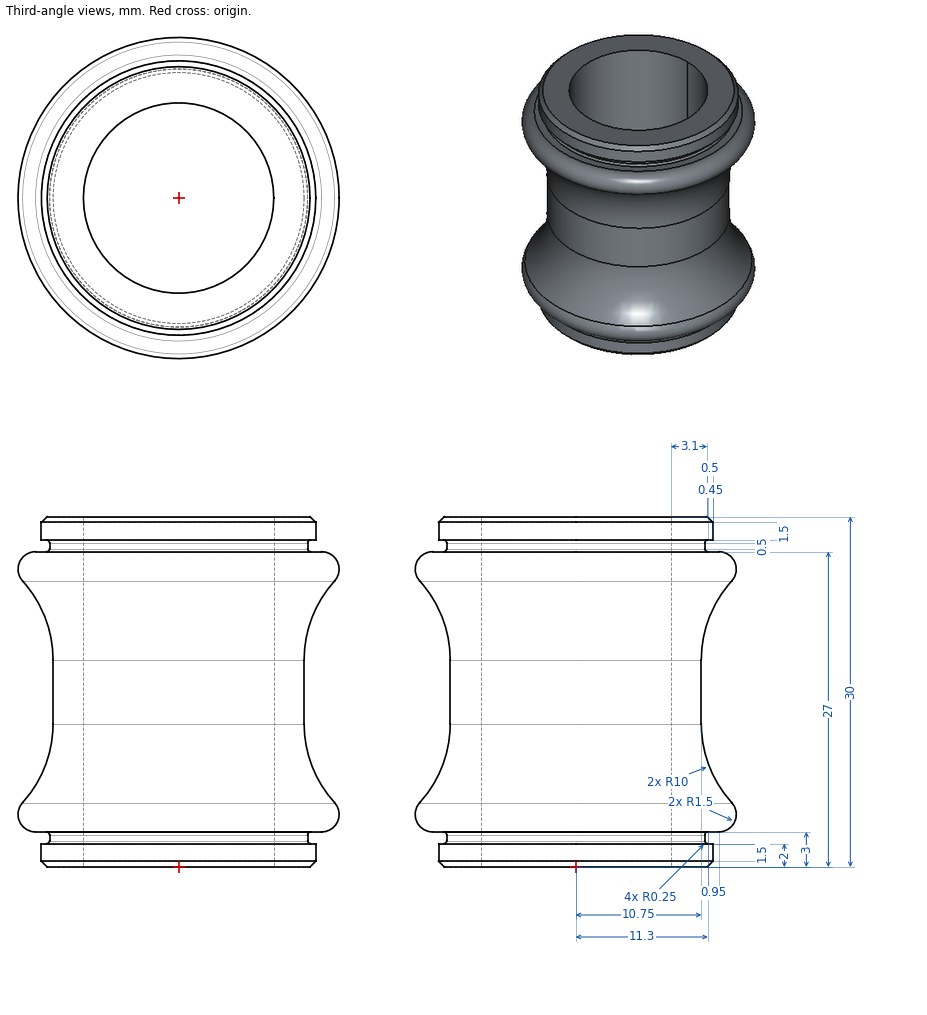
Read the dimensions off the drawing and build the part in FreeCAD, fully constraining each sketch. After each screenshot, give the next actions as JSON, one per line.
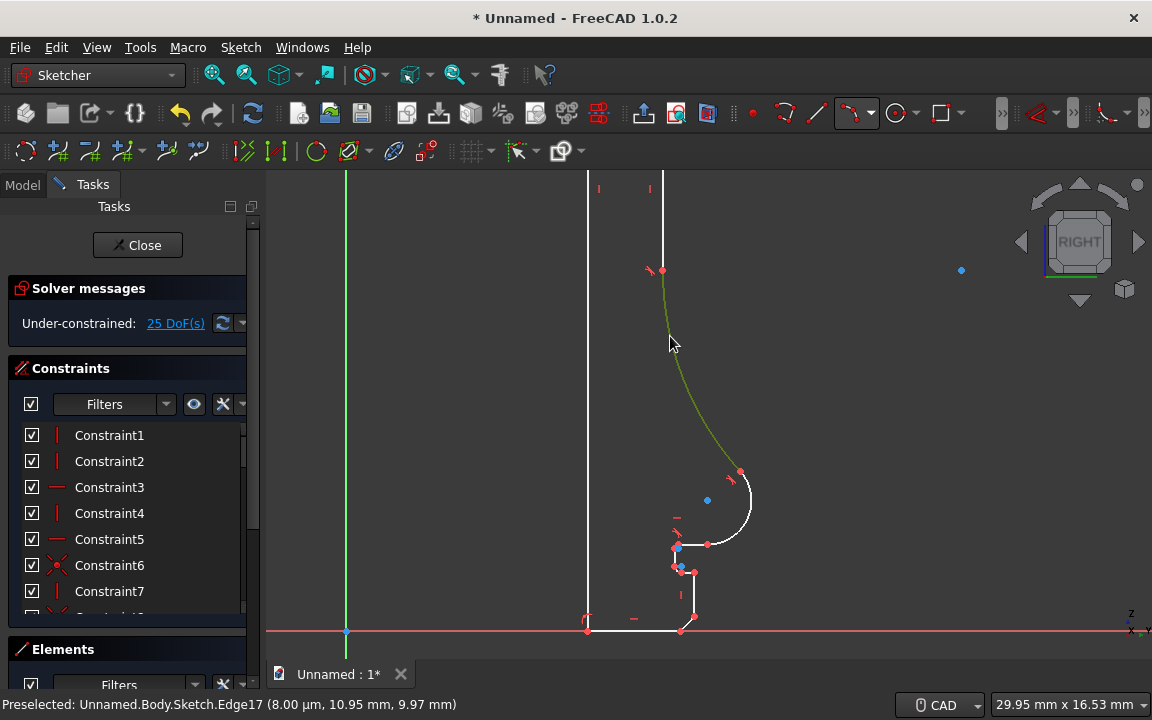
{"action": "scroll", "coordinate": [694, 547], "scroll_direction": "down", "scroll_amount": 5}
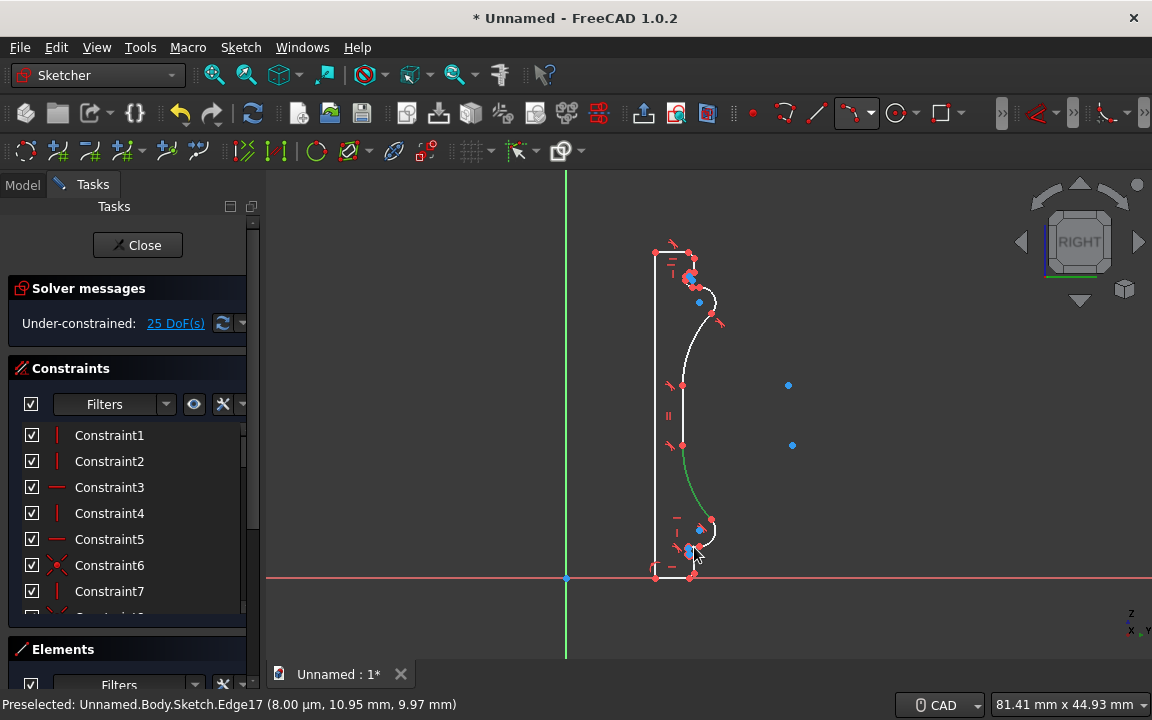
{"action": "left_click", "coordinate": [697, 333]}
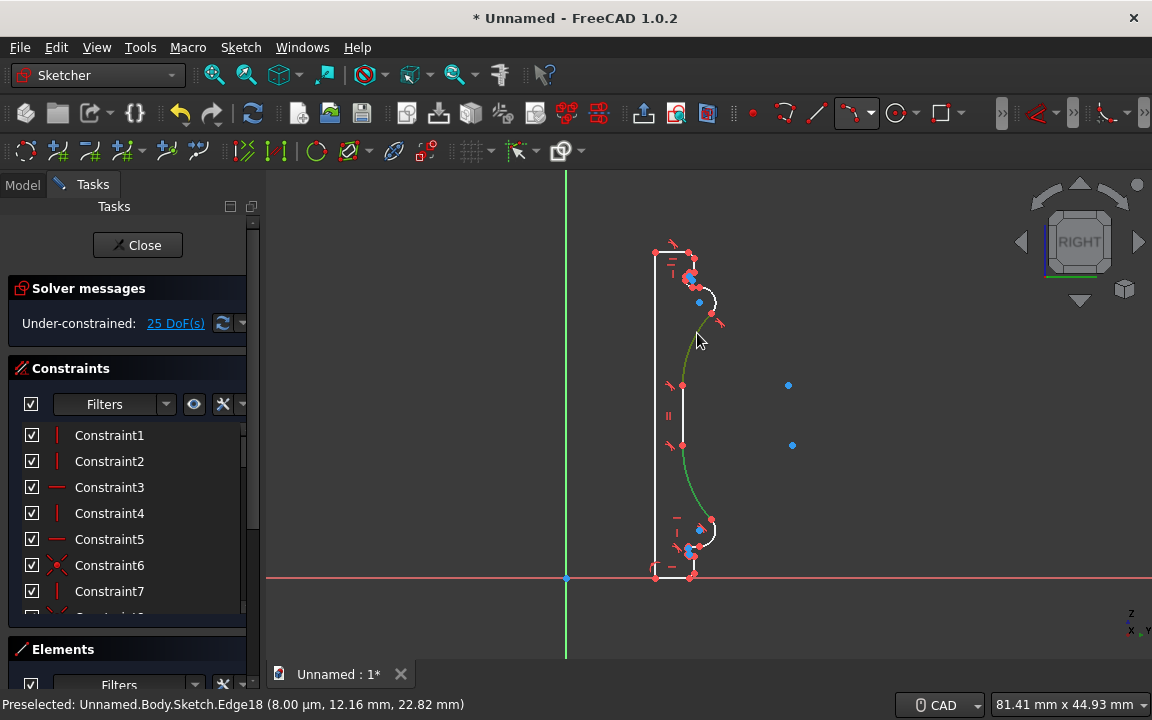
{"action": "key", "text": "e"}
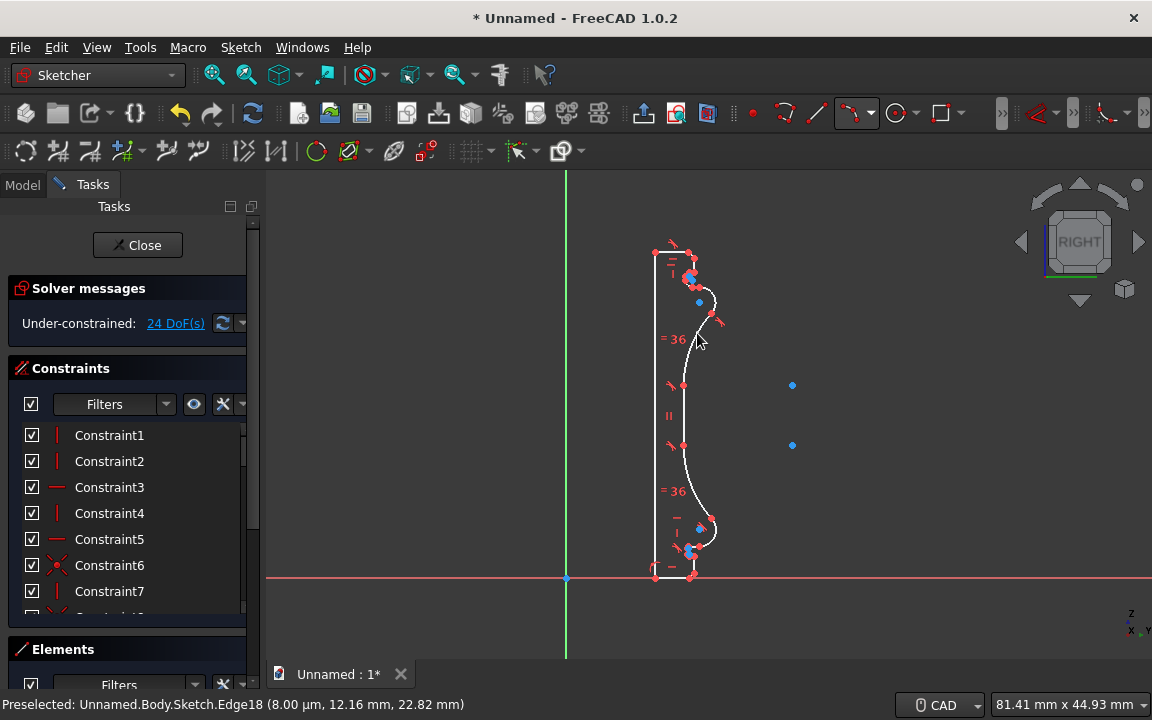
{"action": "left_click", "coordinate": [716, 529]}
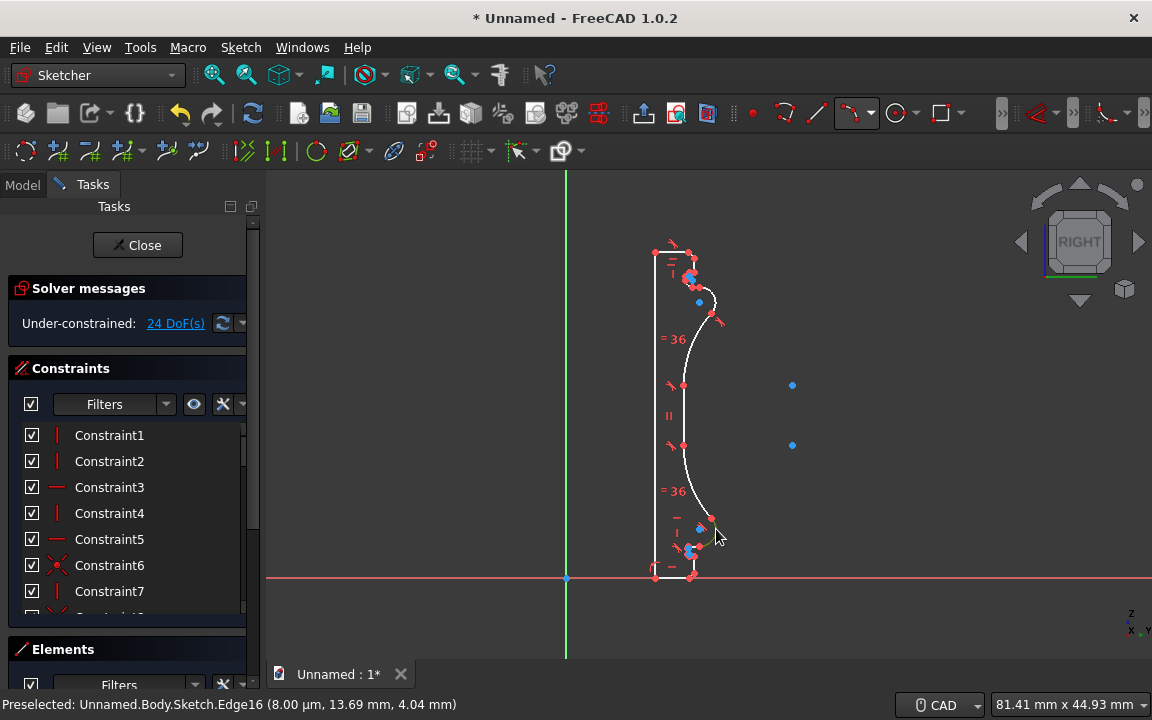
{"action": "scroll", "coordinate": [716, 303], "scroll_direction": "up", "scroll_amount": 2}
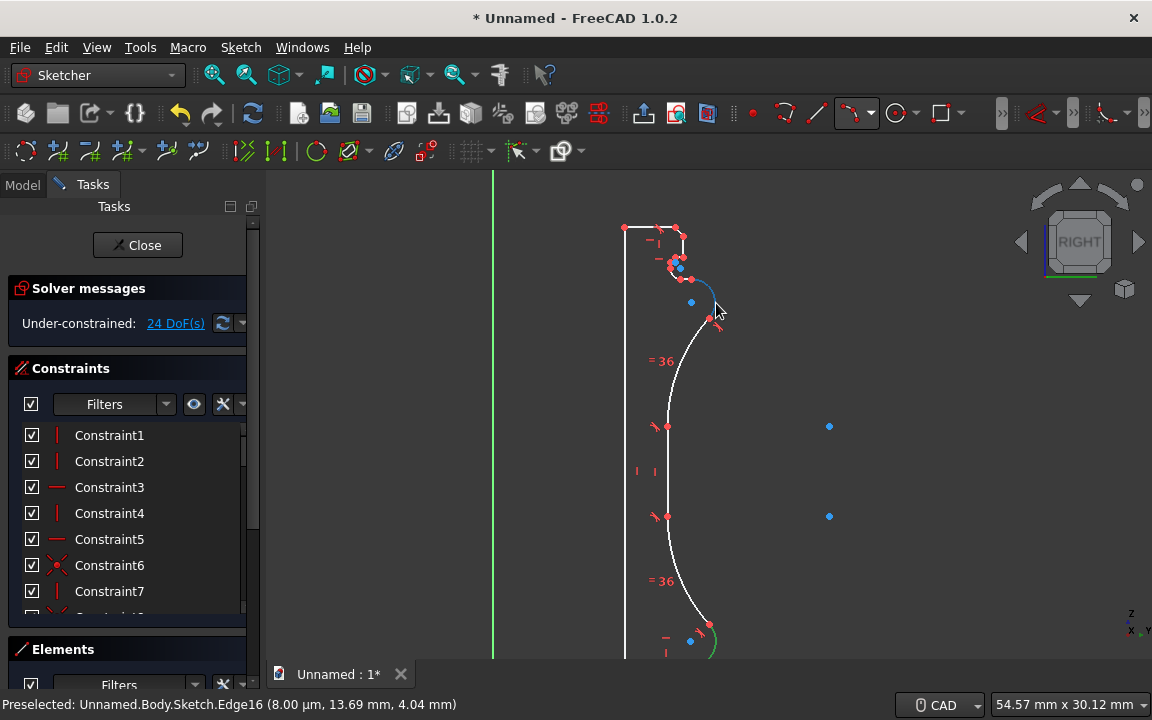
{"action": "left_click", "coordinate": [715, 304]}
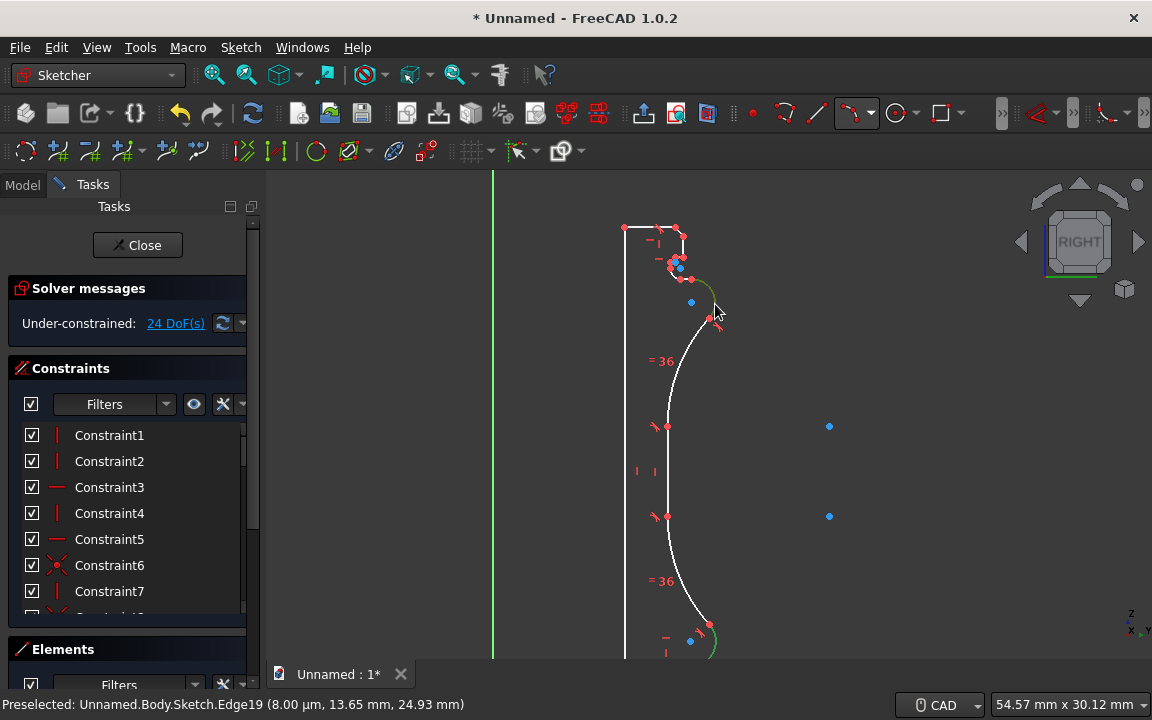
{"action": "key", "text": "e"}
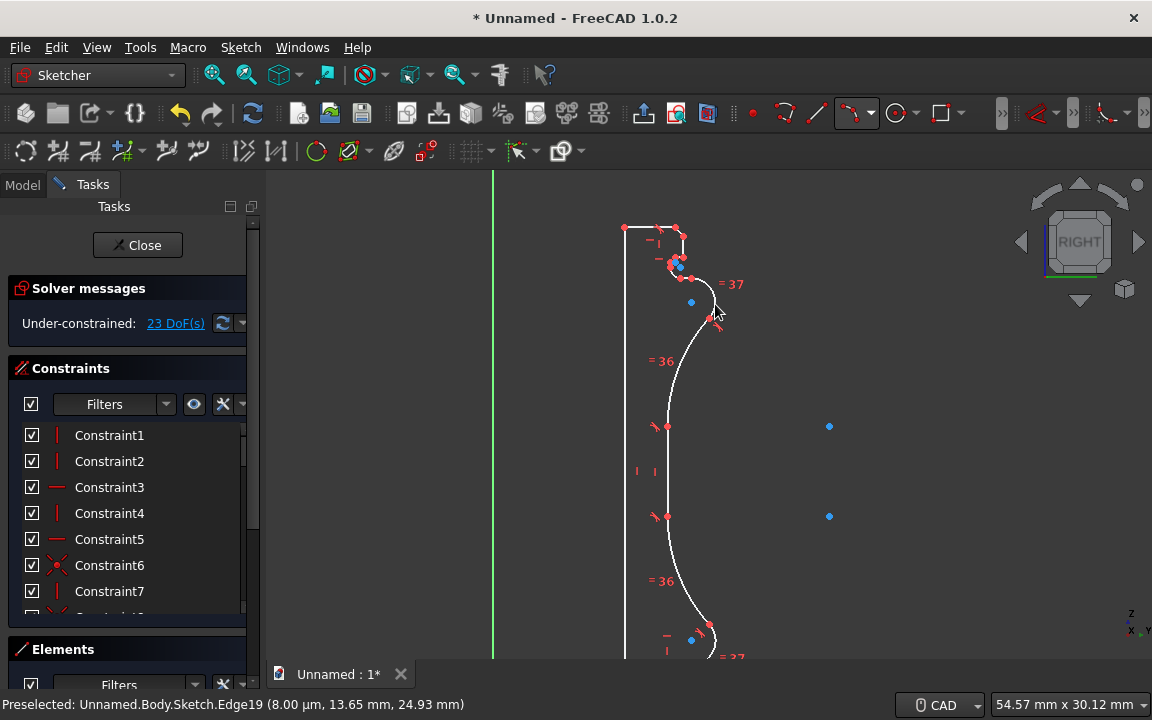
{"action": "scroll", "coordinate": [716, 301], "scroll_direction": "down", "scroll_amount": 2}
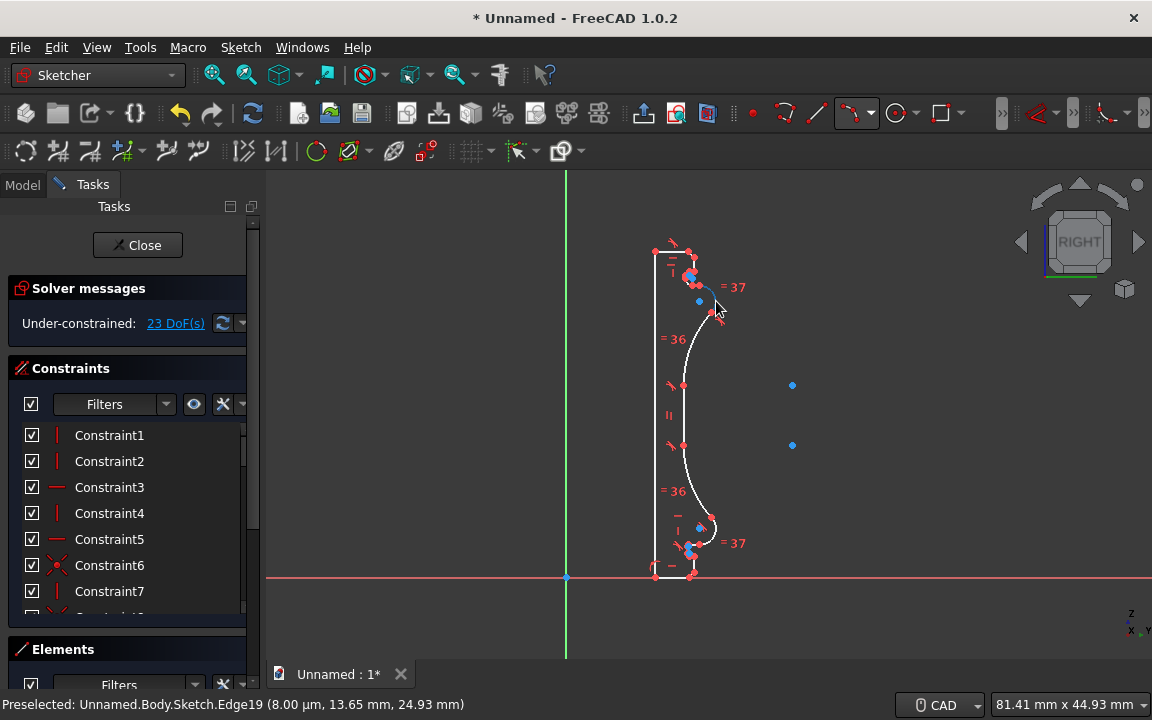
{"action": "scroll", "coordinate": [688, 545], "scroll_direction": "up", "scroll_amount": 13}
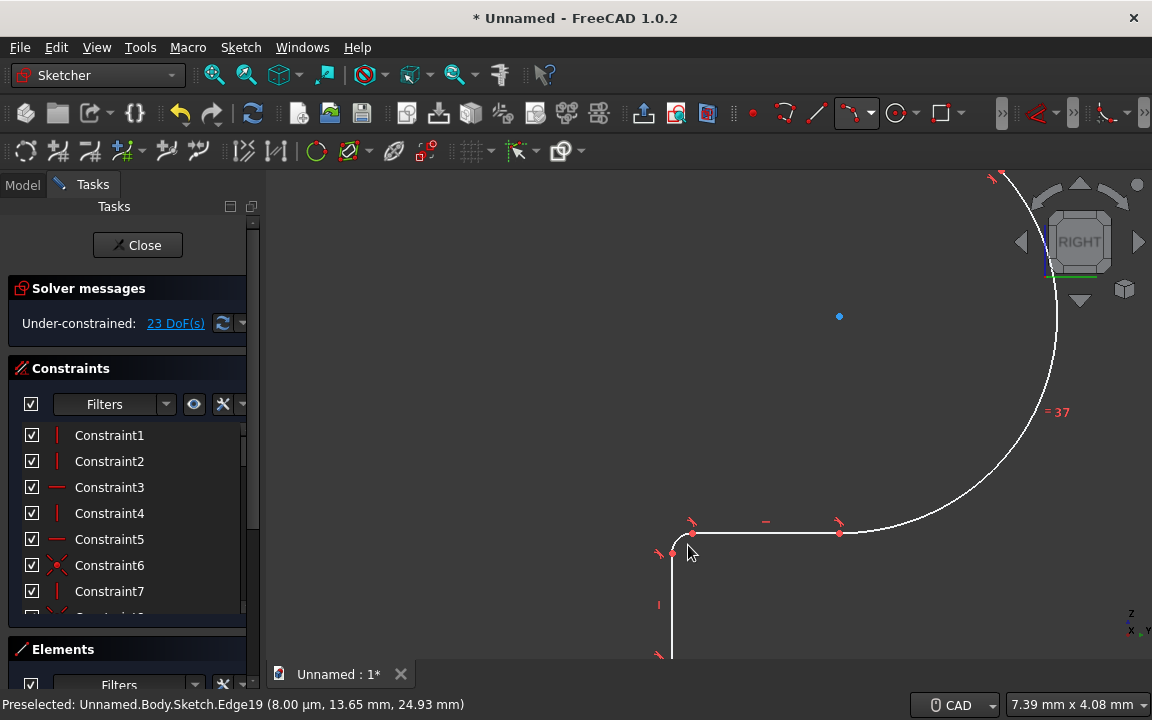
{"action": "left_click", "coordinate": [678, 539]}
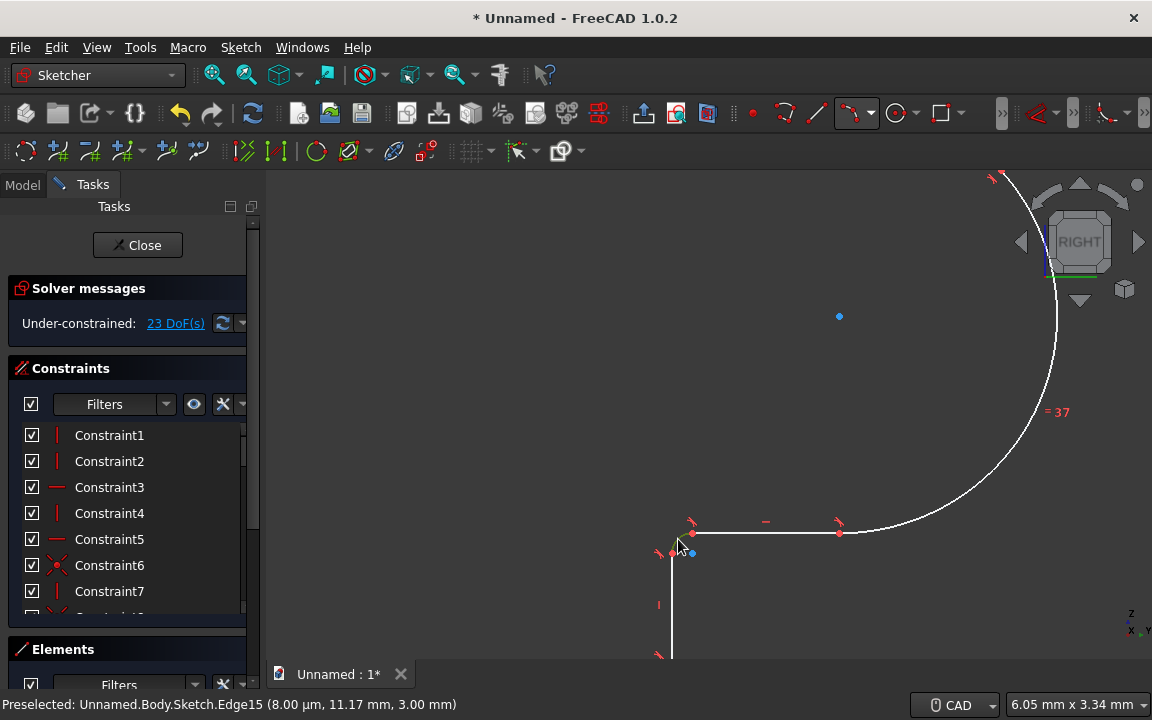
{"action": "scroll", "coordinate": [688, 546], "scroll_direction": "down", "scroll_amount": 13}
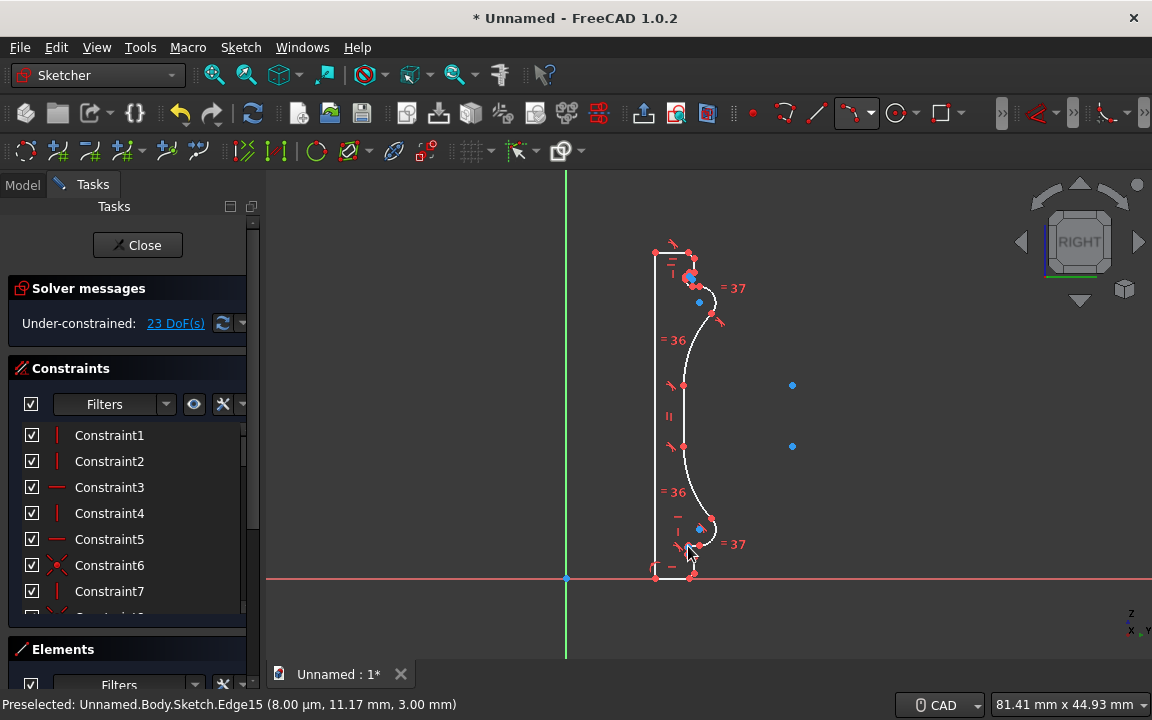
{"action": "scroll", "coordinate": [686, 283], "scroll_direction": "up", "scroll_amount": 8}